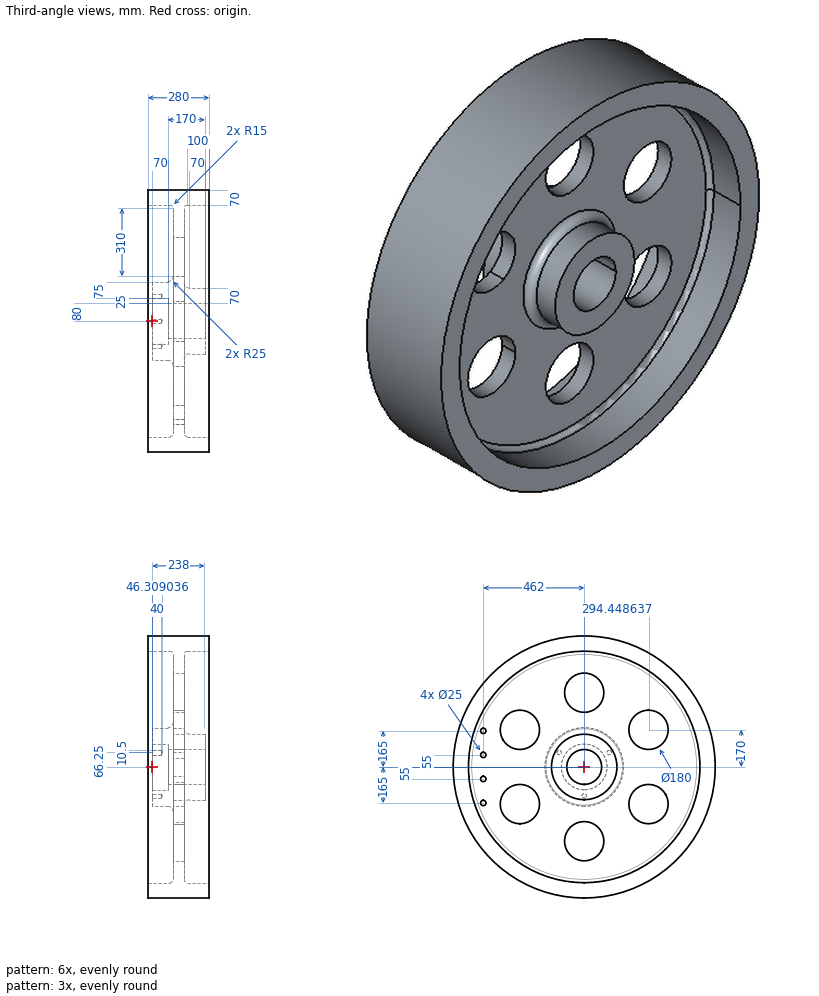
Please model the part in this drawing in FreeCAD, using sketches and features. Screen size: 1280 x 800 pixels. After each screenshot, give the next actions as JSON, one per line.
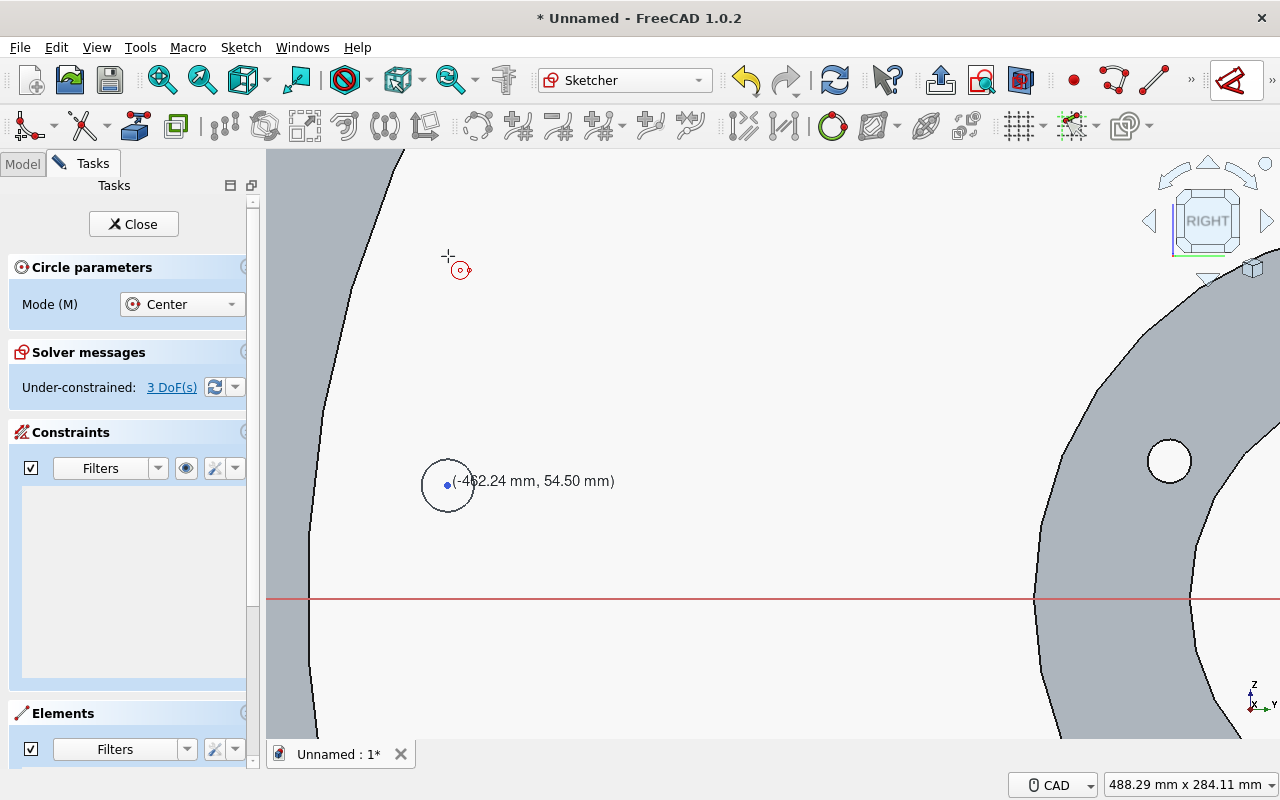
{"action": "left_click", "coordinate": [448, 256]}
{"action": "left_click", "coordinate": [467, 238]}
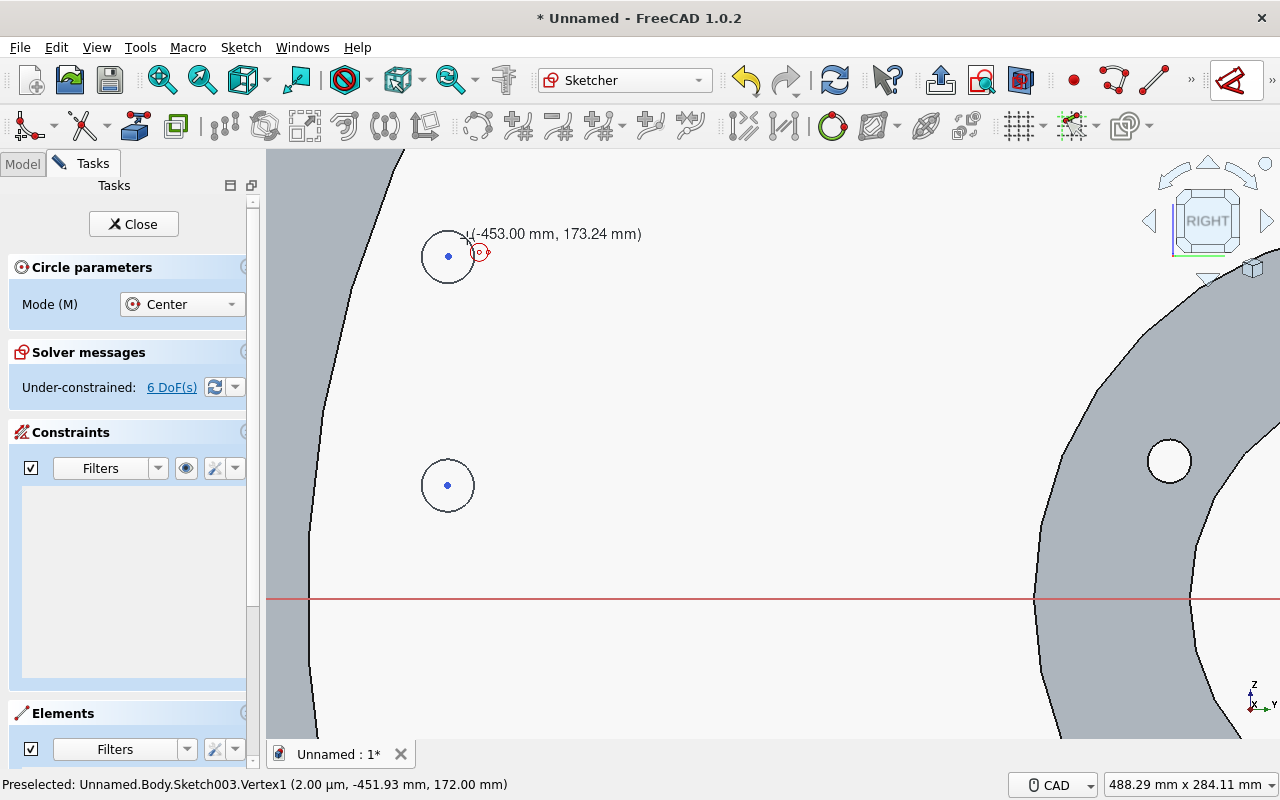
{"action": "scroll", "coordinate": [448, 256], "scroll_direction": "down", "scroll_amount": 3}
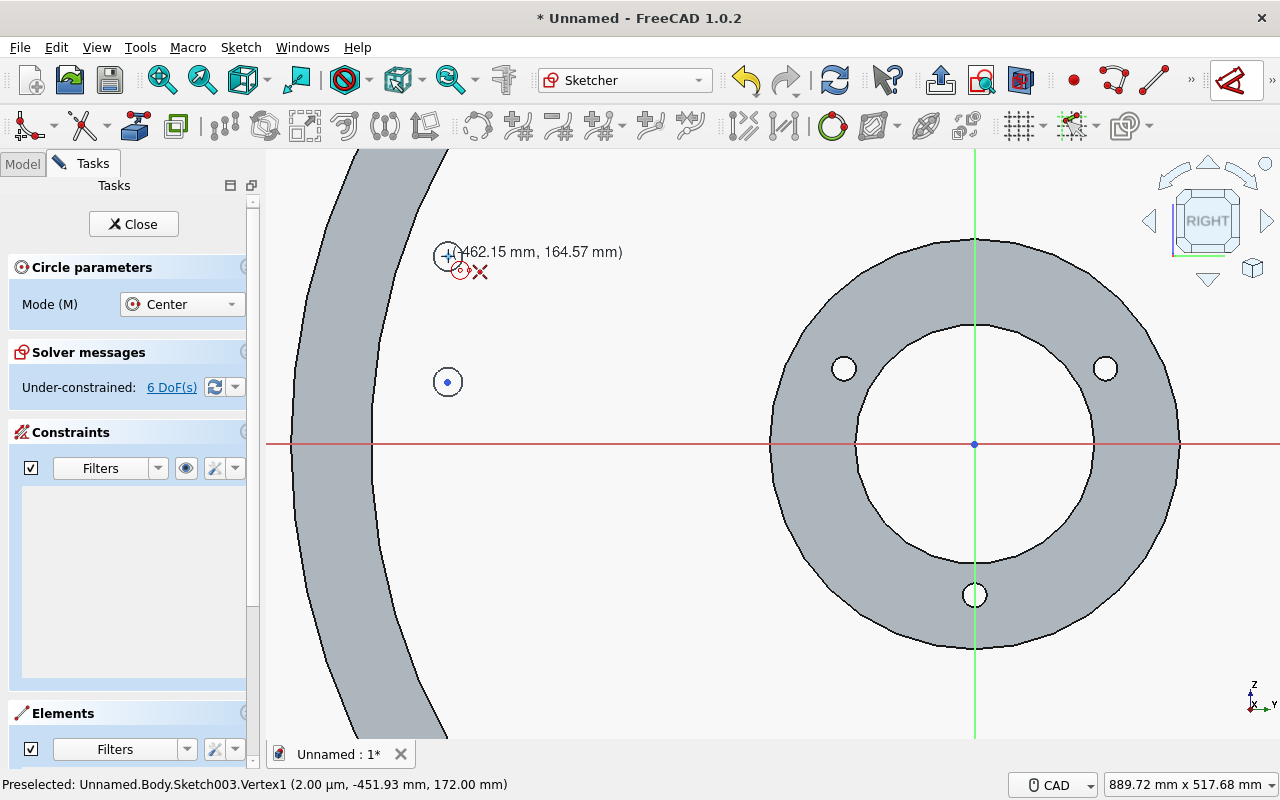
{"action": "scroll", "coordinate": [448, 507], "scroll_direction": "up", "scroll_amount": 3}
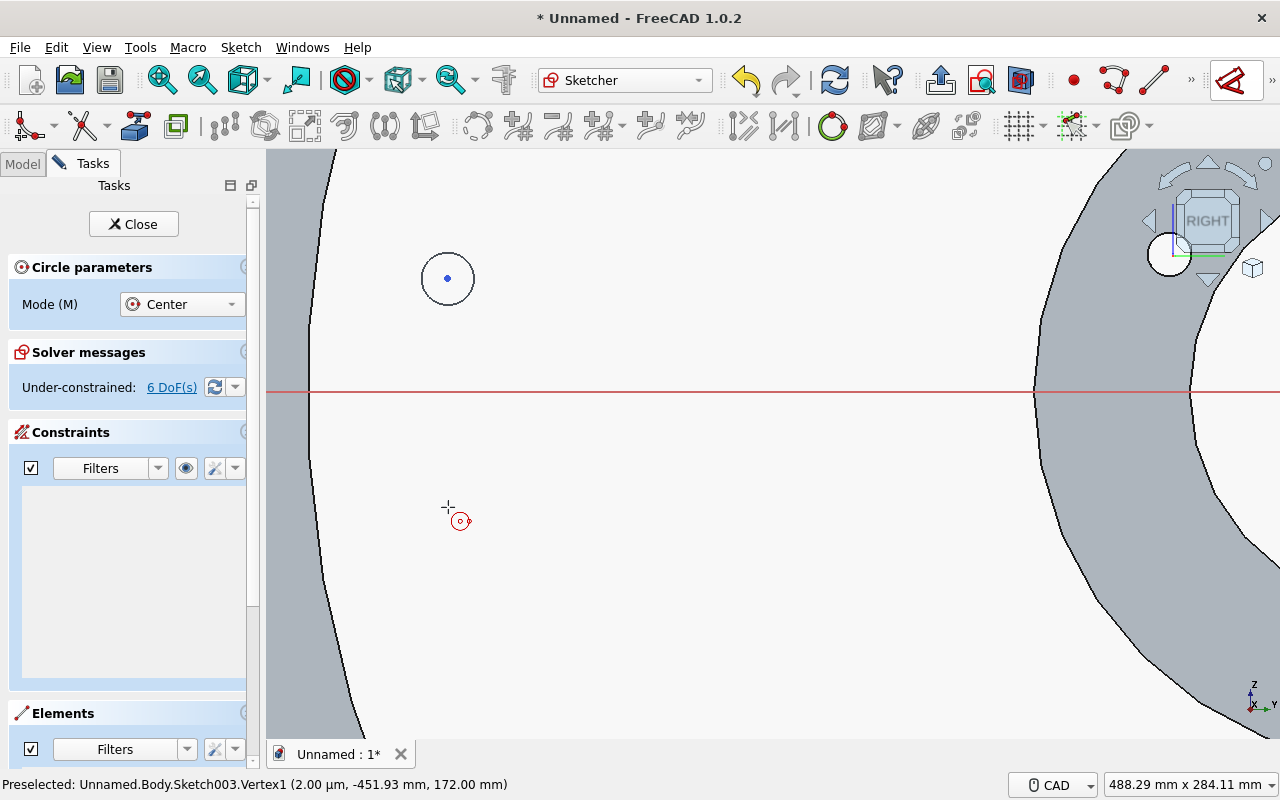
{"action": "left_click", "coordinate": [448, 506]}
{"action": "left_click", "coordinate": [467, 488]}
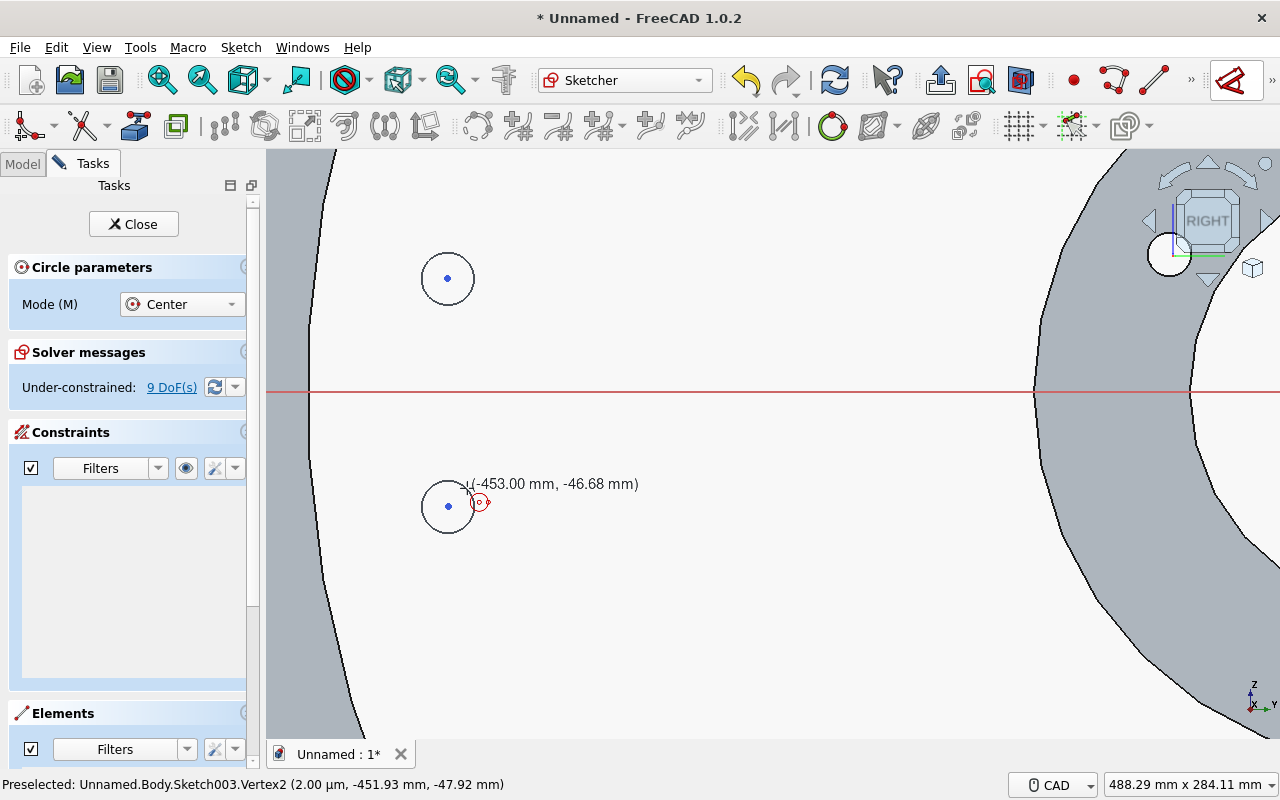
{"action": "scroll", "coordinate": [448, 507], "scroll_direction": "down", "scroll_amount": 3}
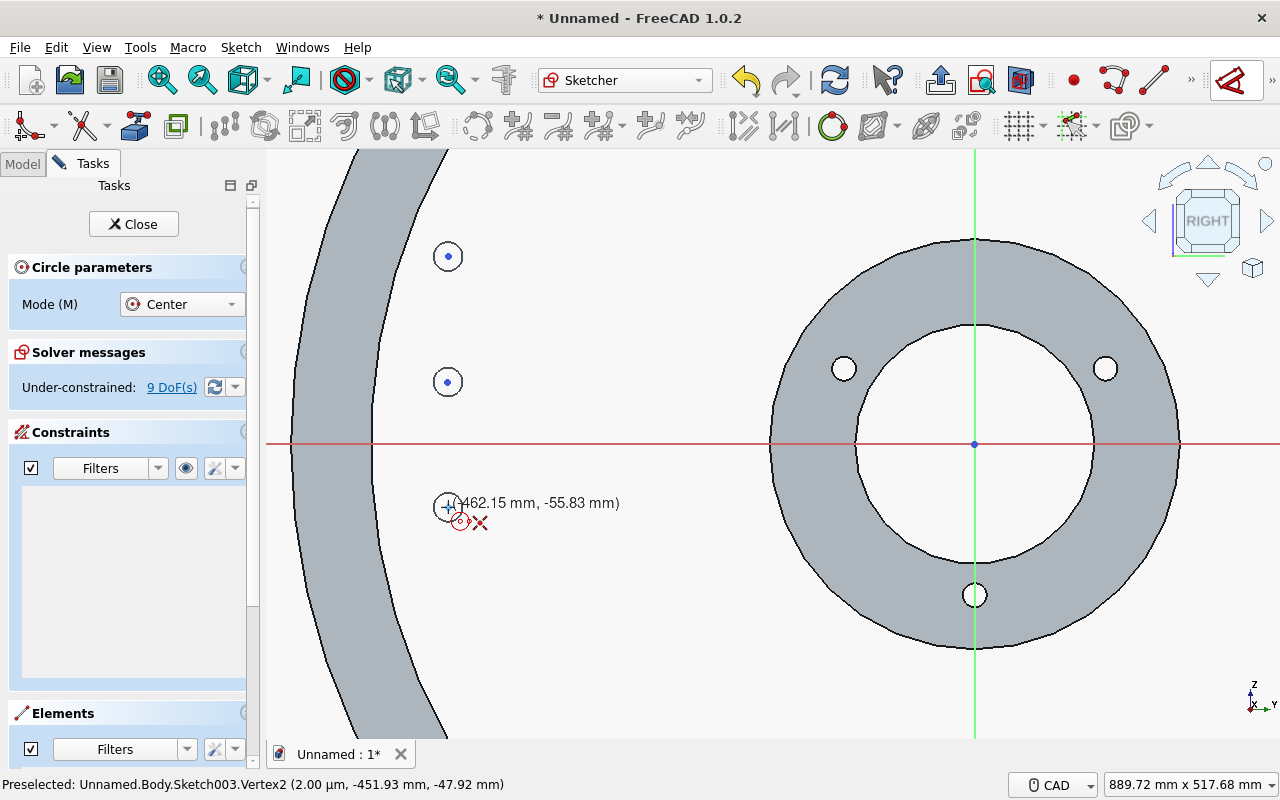
{"action": "scroll", "coordinate": [448, 632], "scroll_direction": "up", "scroll_amount": 3}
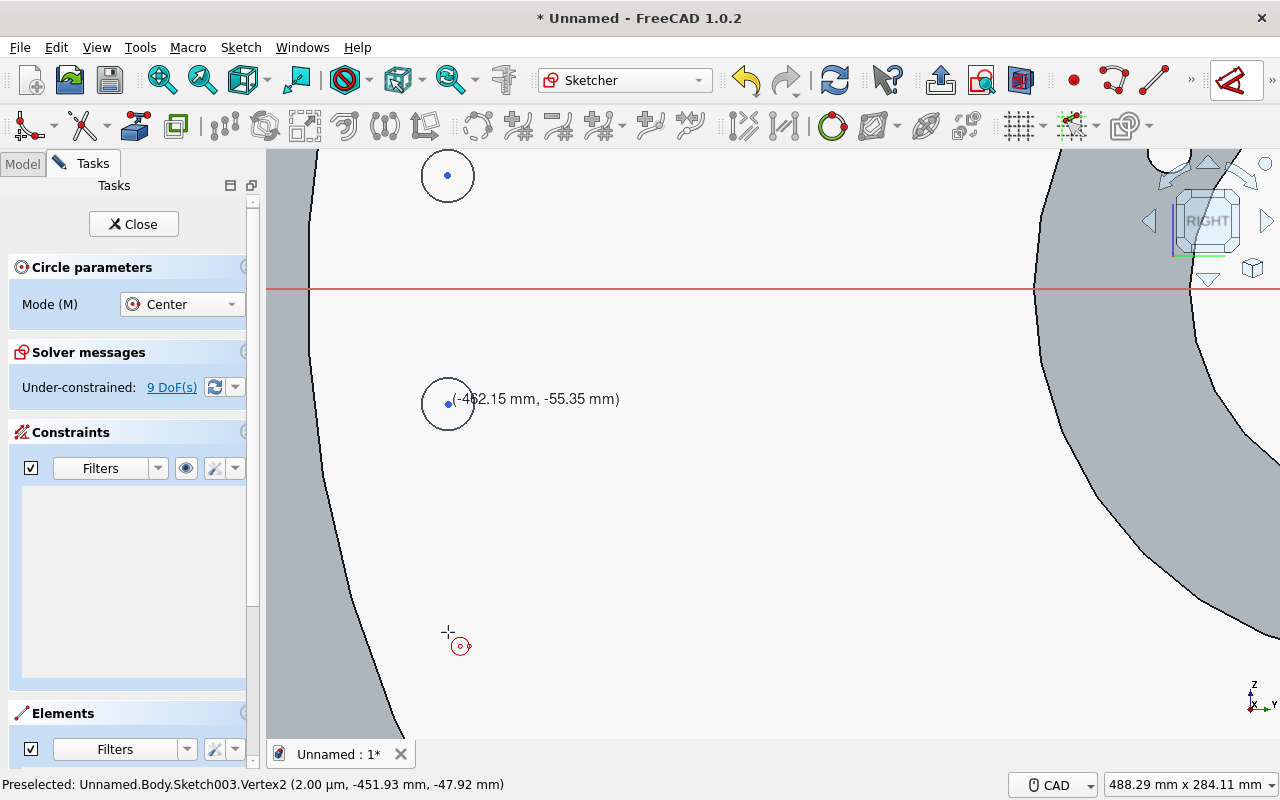
{"action": "left_click", "coordinate": [448, 632]}
{"action": "left_click", "coordinate": [467, 613]}
{"action": "key", "text": "Escape"}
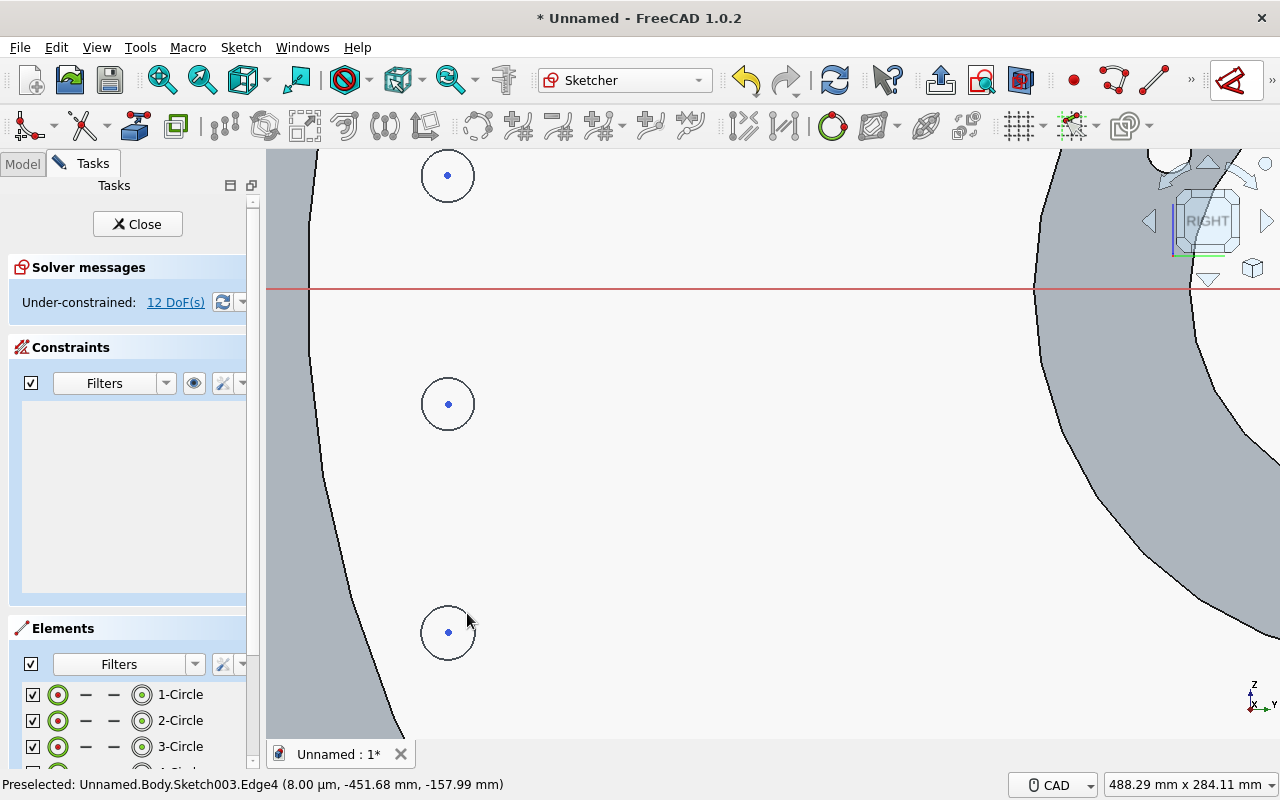
{"action": "left_click", "coordinate": [429, 195]}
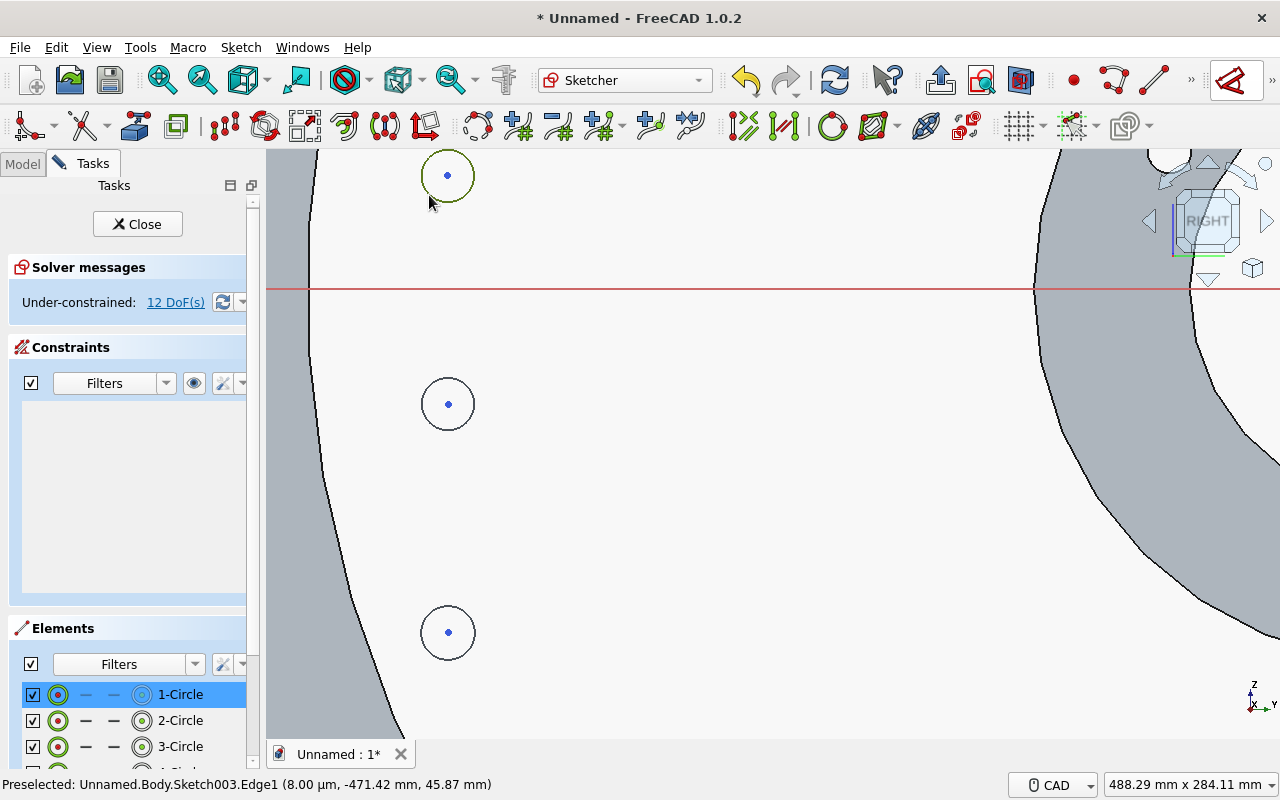
{"action": "scroll", "coordinate": [448, 632], "scroll_direction": "down", "scroll_amount": 3}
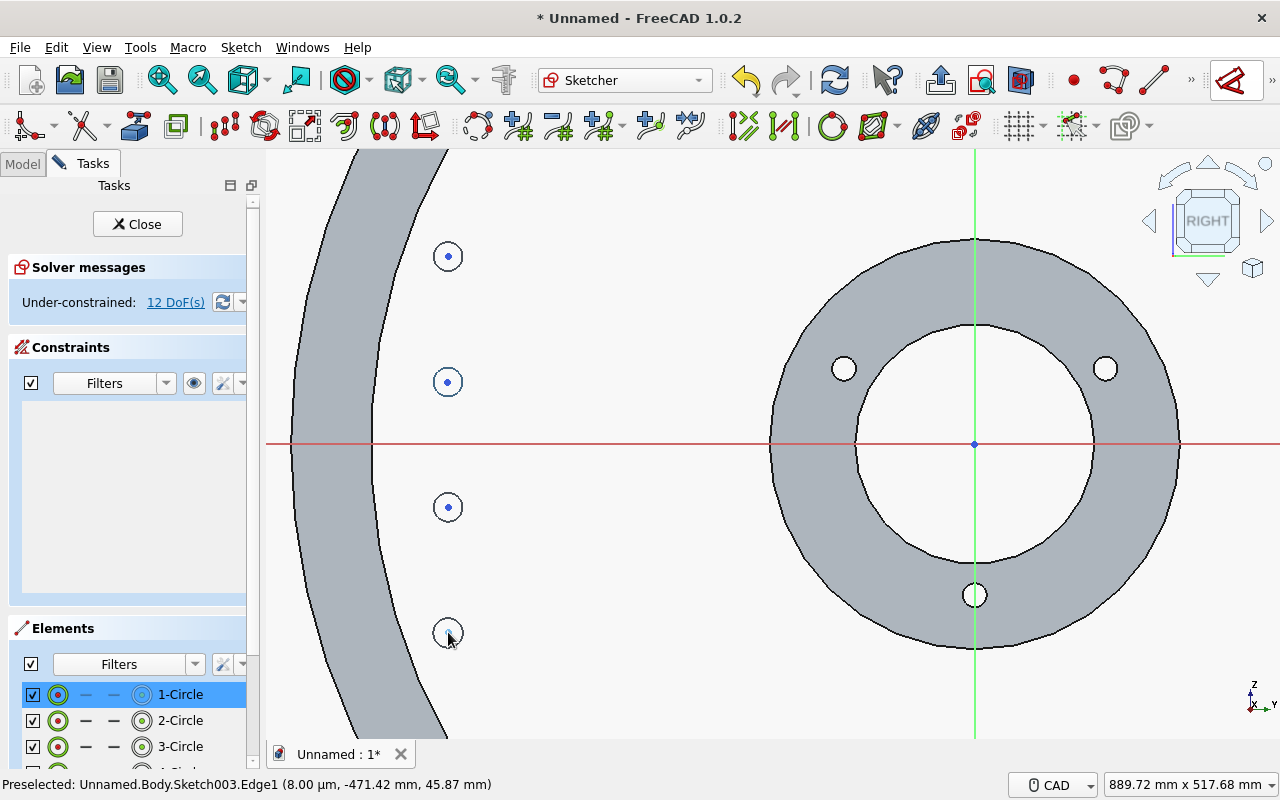
{"action": "left_click", "coordinate": [458, 246]}